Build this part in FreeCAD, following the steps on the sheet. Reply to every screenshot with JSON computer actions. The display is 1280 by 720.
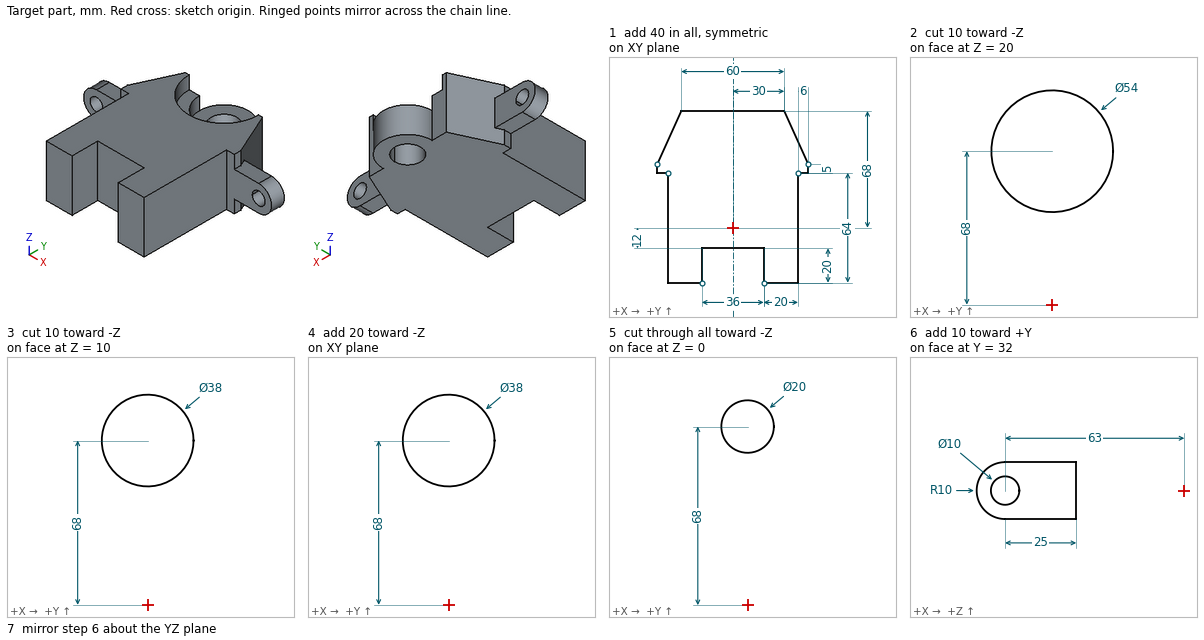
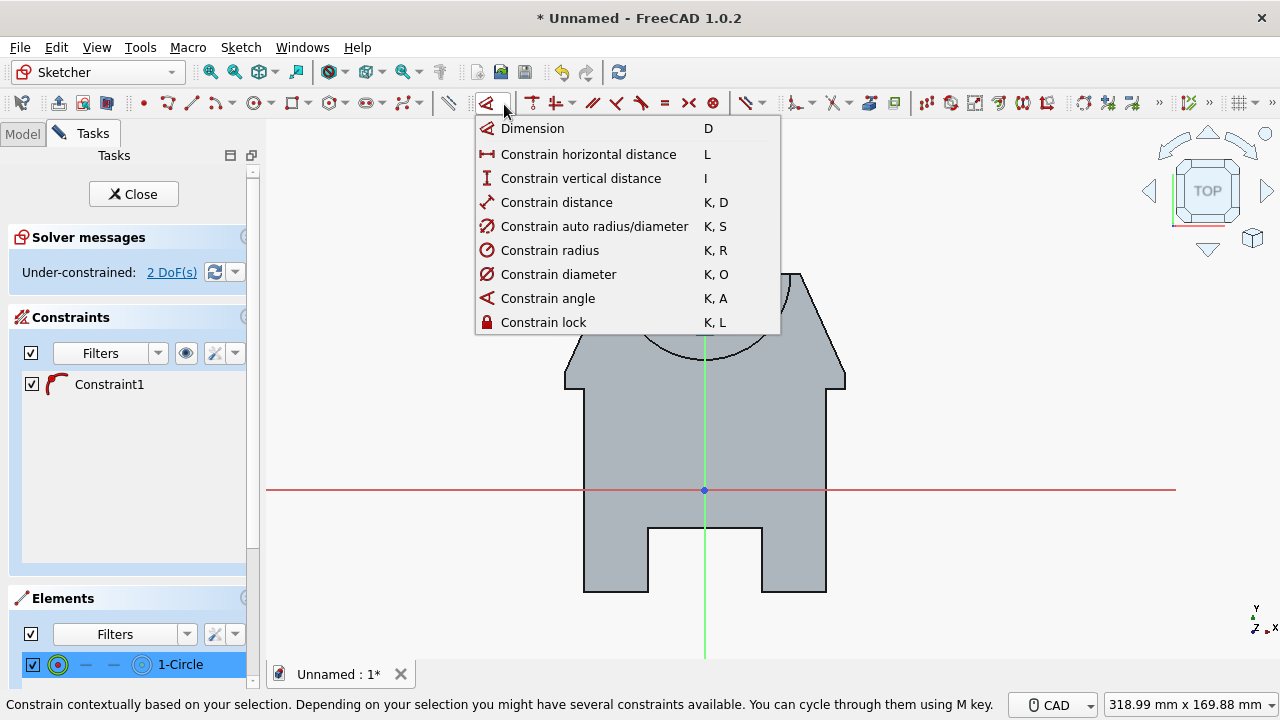
{"action": "left_click", "coordinate": [628, 274]}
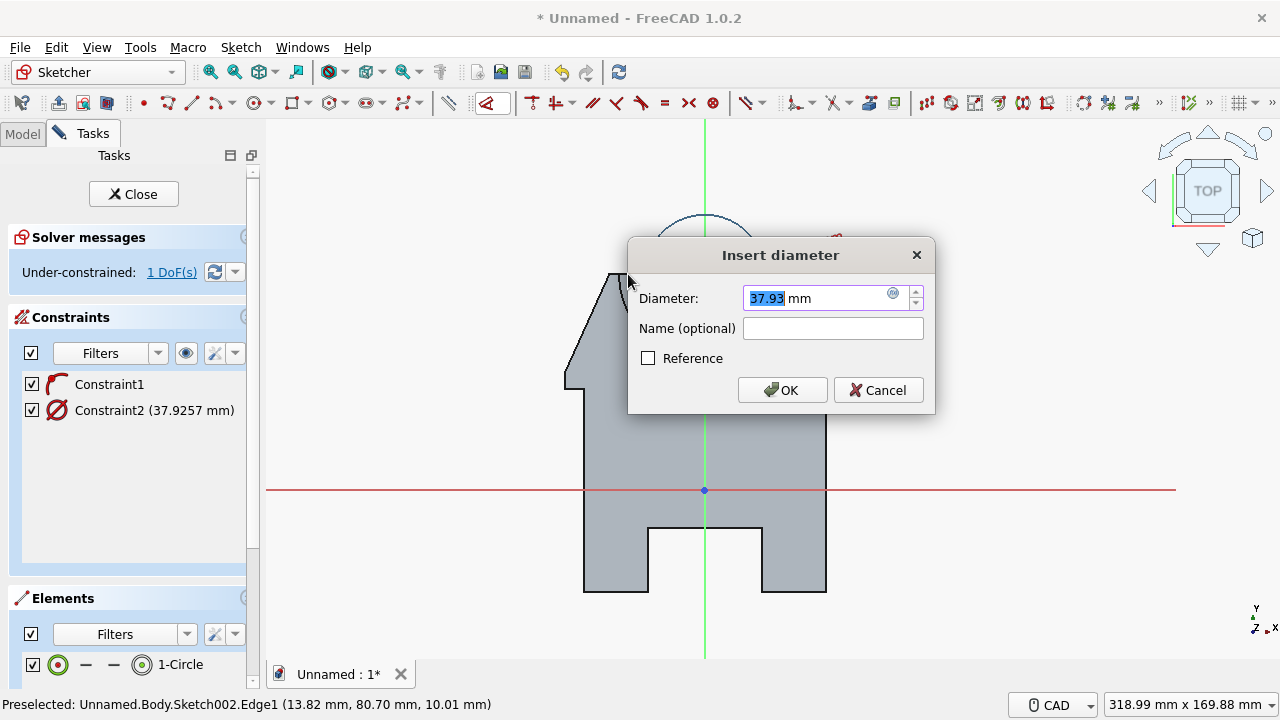
{"action": "type", "text": "38"}
{"action": "key", "text": "Return"}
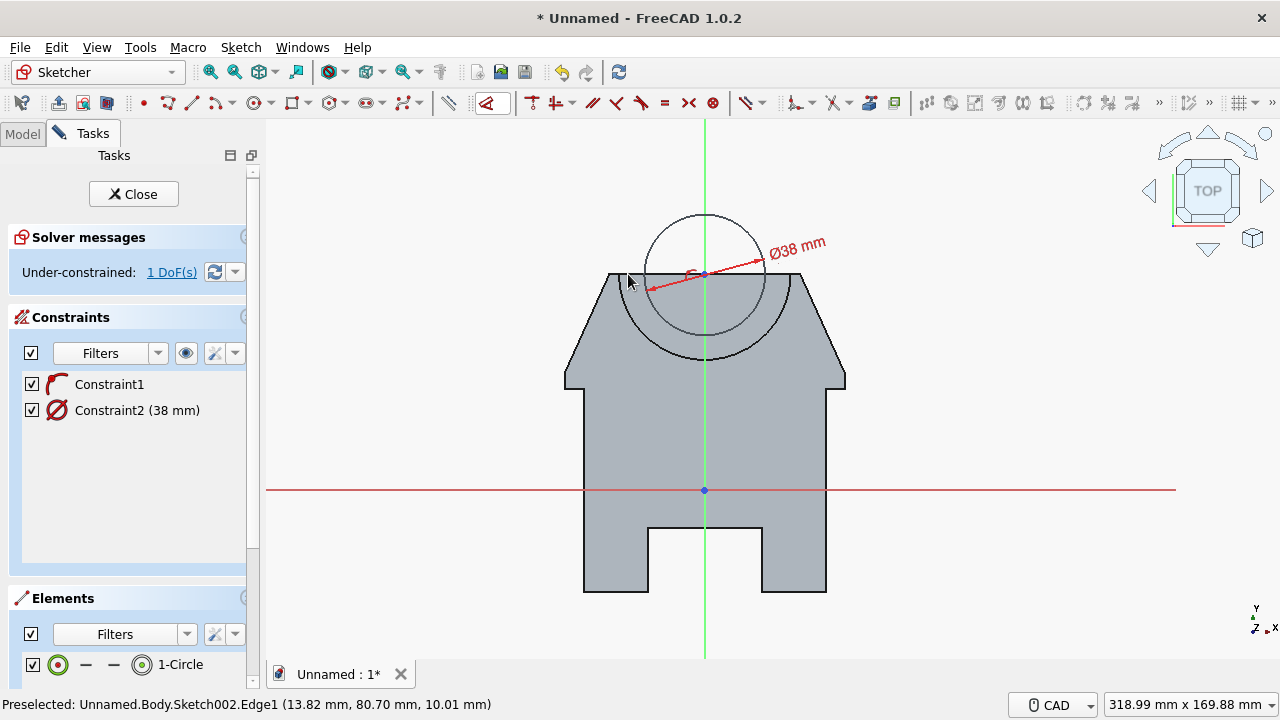
{"action": "left_click", "coordinate": [705, 275]}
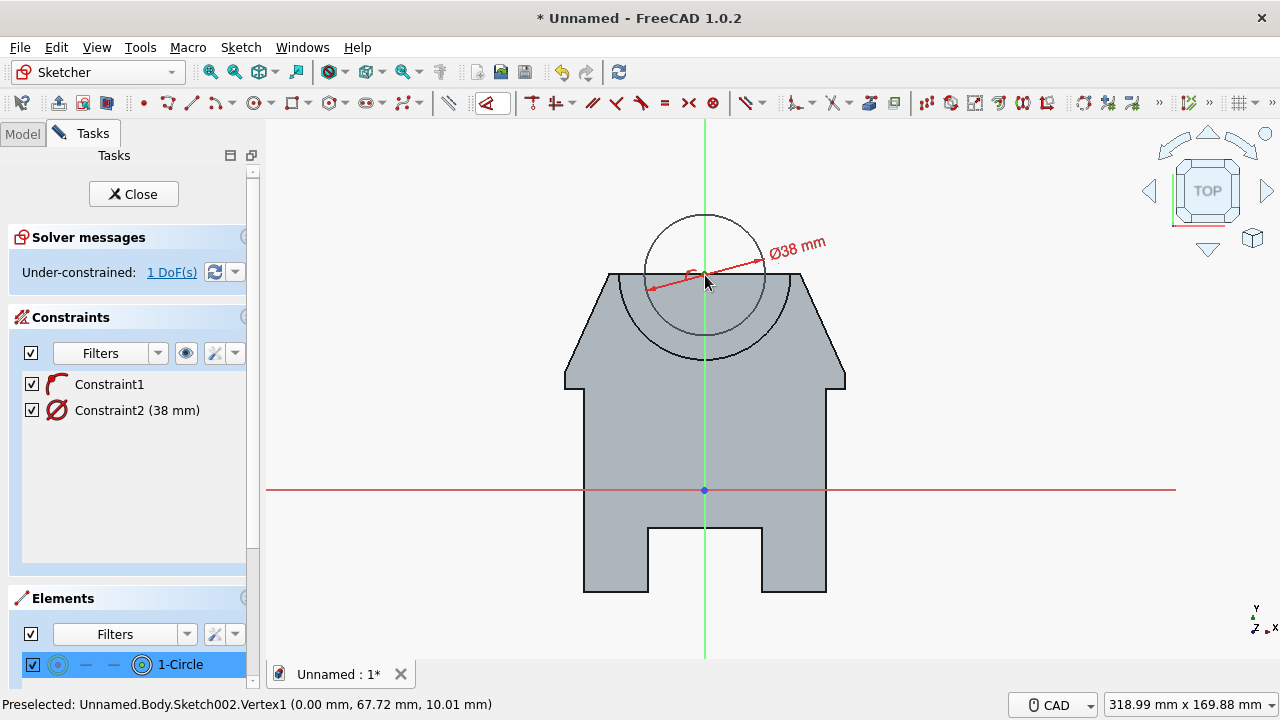
{"action": "key", "text": "i"}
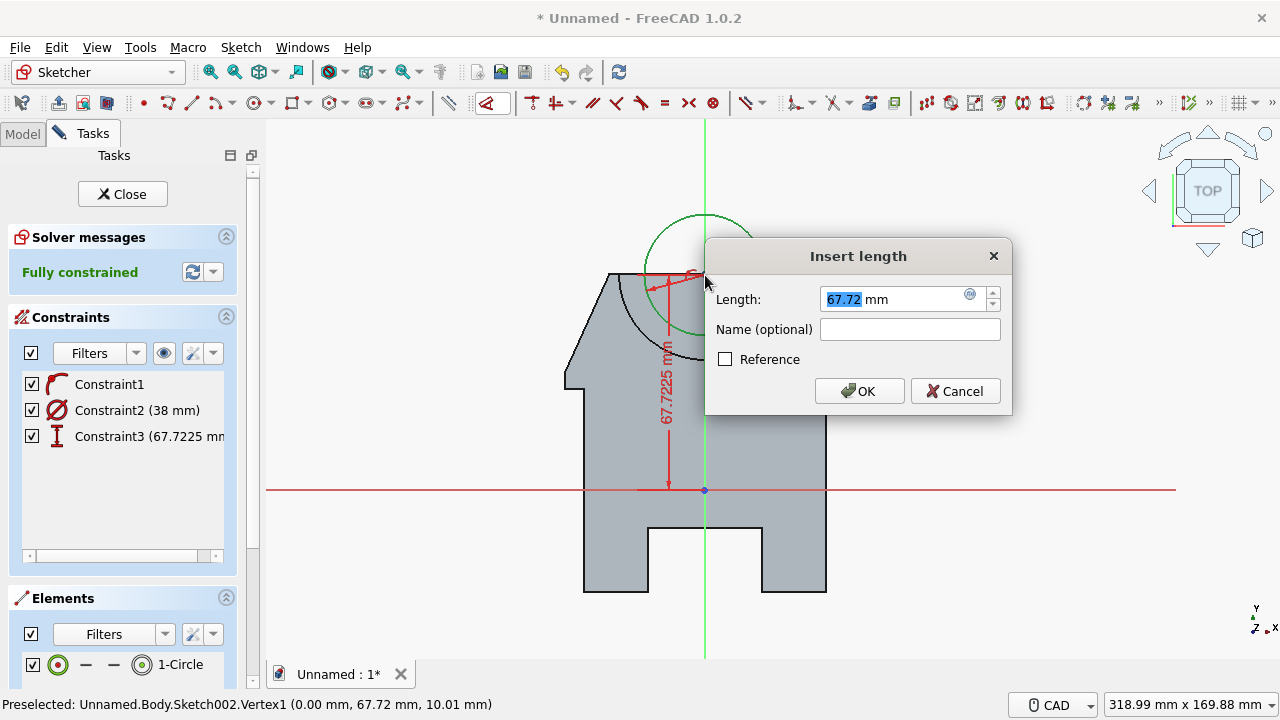
{"action": "type", "text": "68"}
{"action": "key", "text": "Return"}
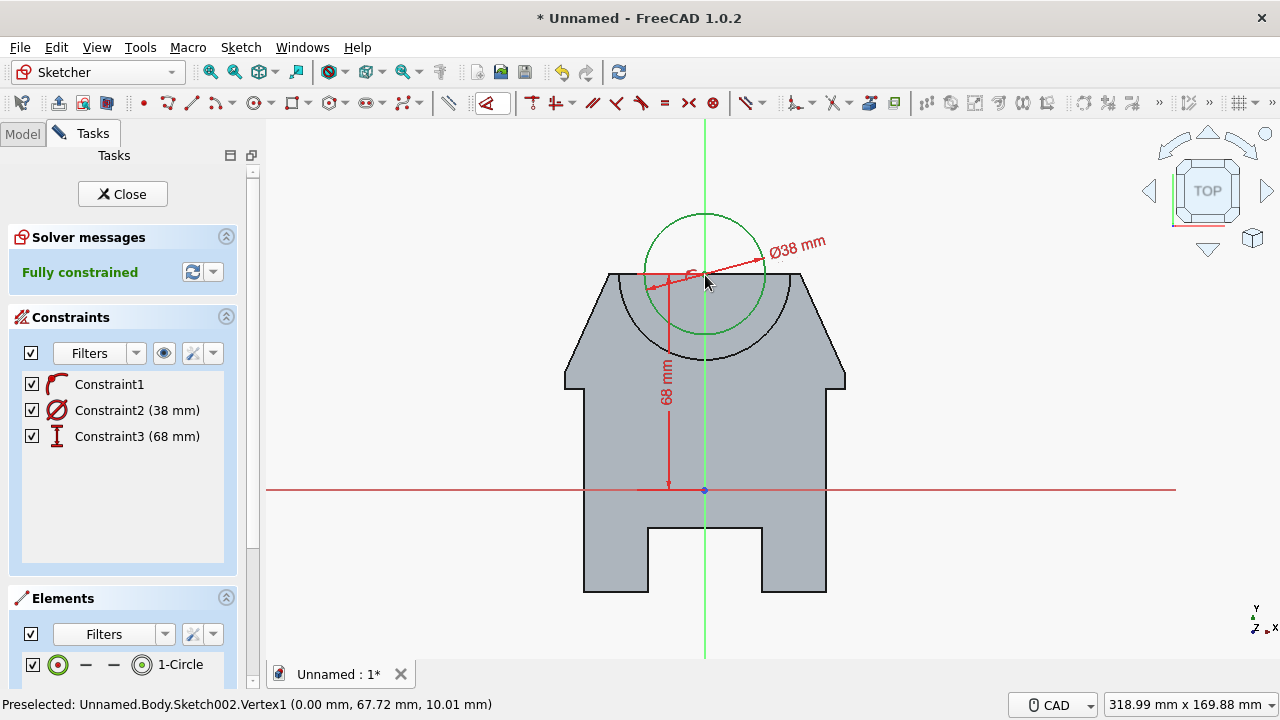
{"action": "left_click", "coordinate": [123, 194]}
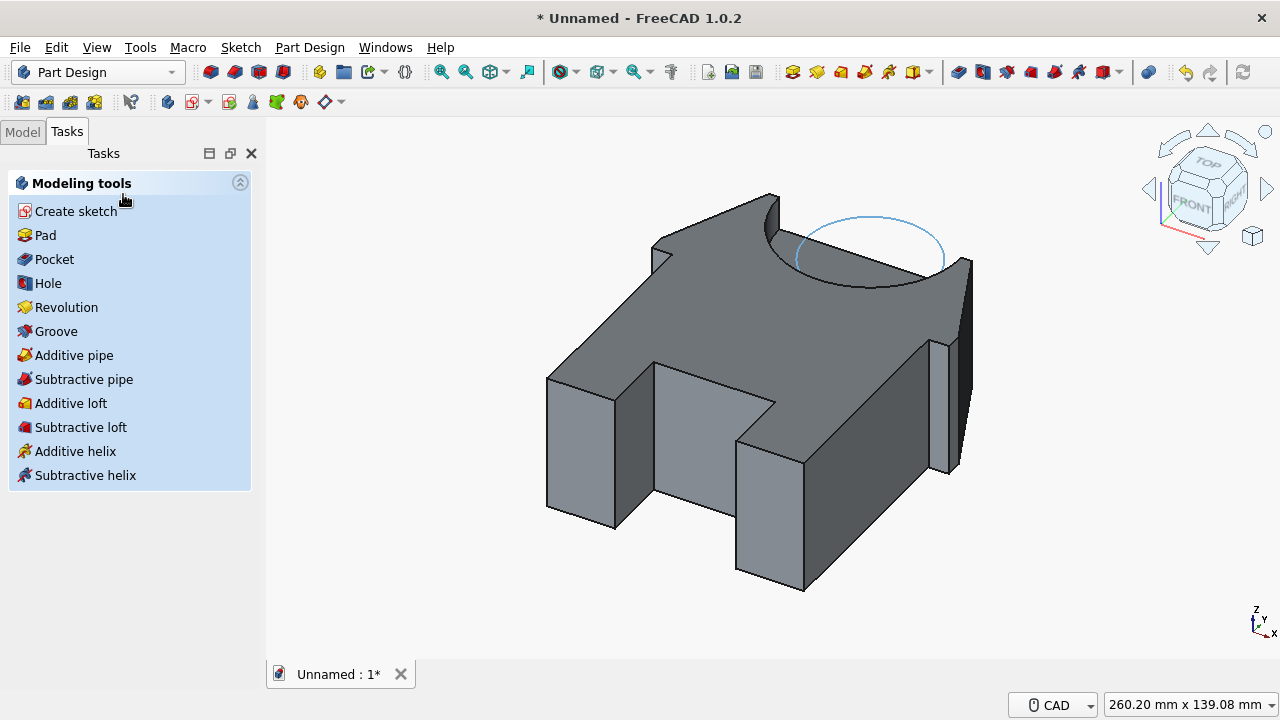
{"action": "left_click", "coordinate": [960, 72]}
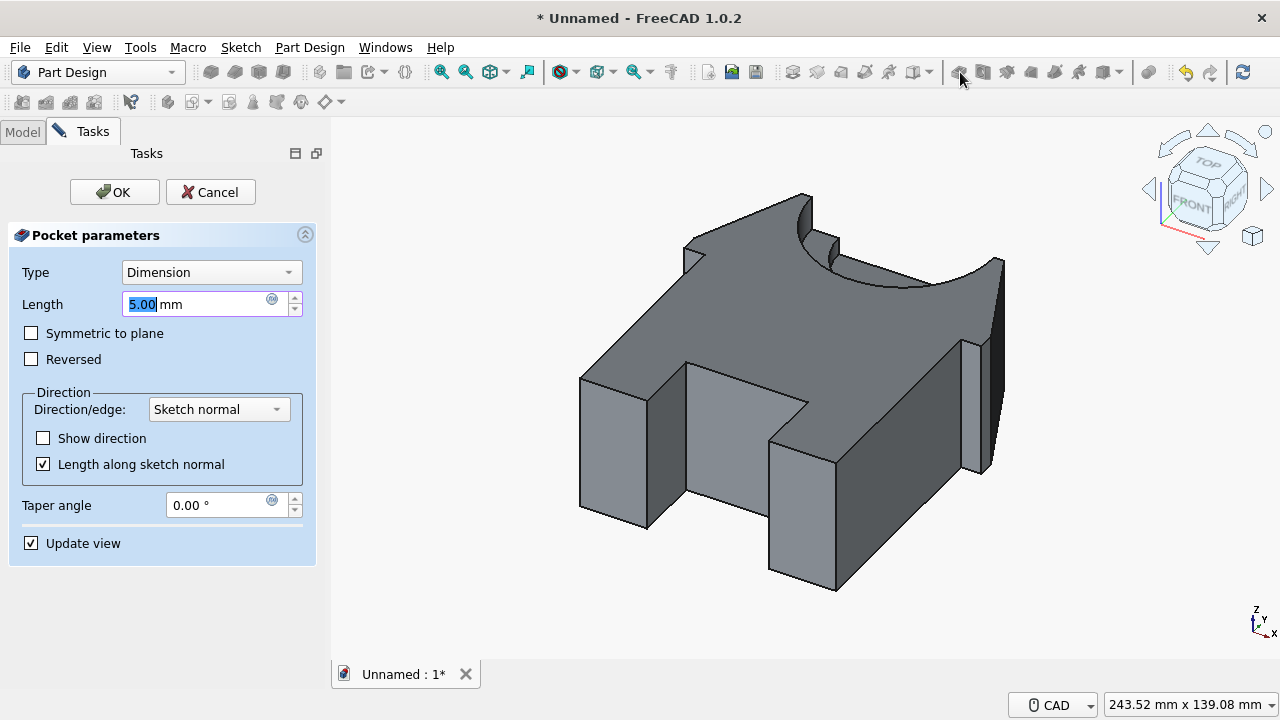
{"action": "type", "text": "10"}
{"action": "key", "text": "Tab"}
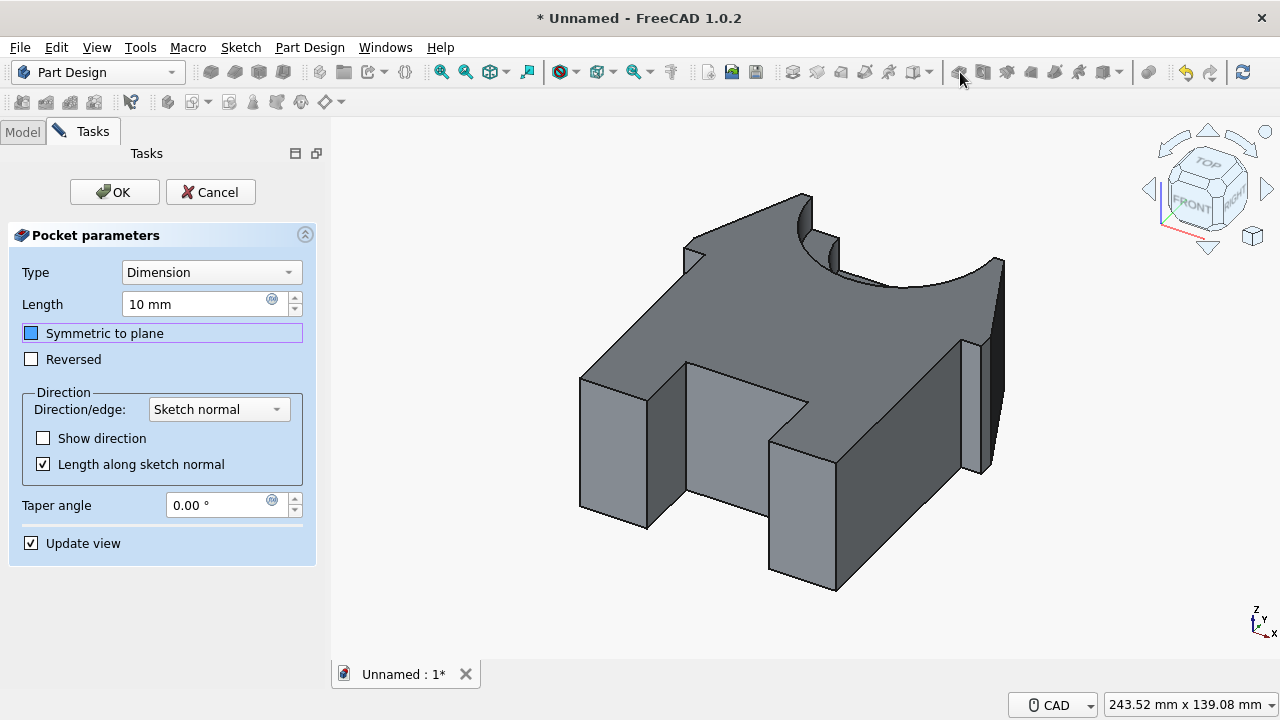
{"action": "left_click", "coordinate": [115, 192]}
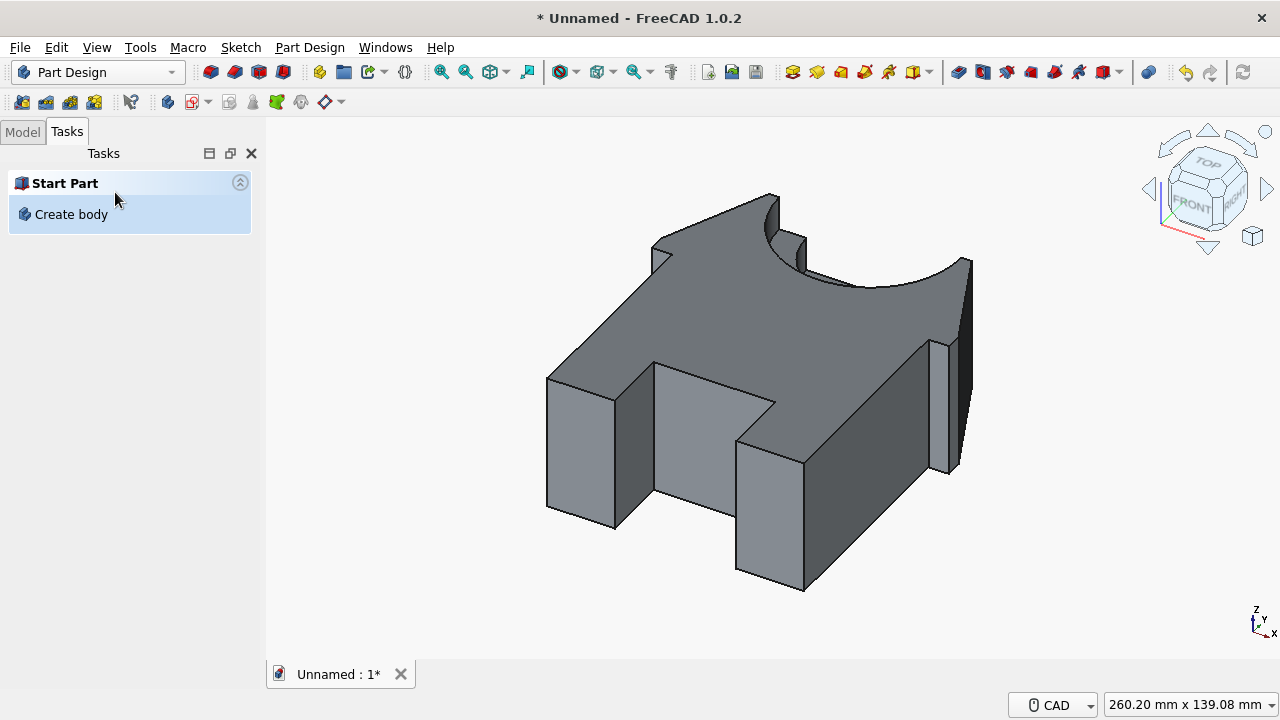
{"action": "left_click", "coordinate": [192, 102]}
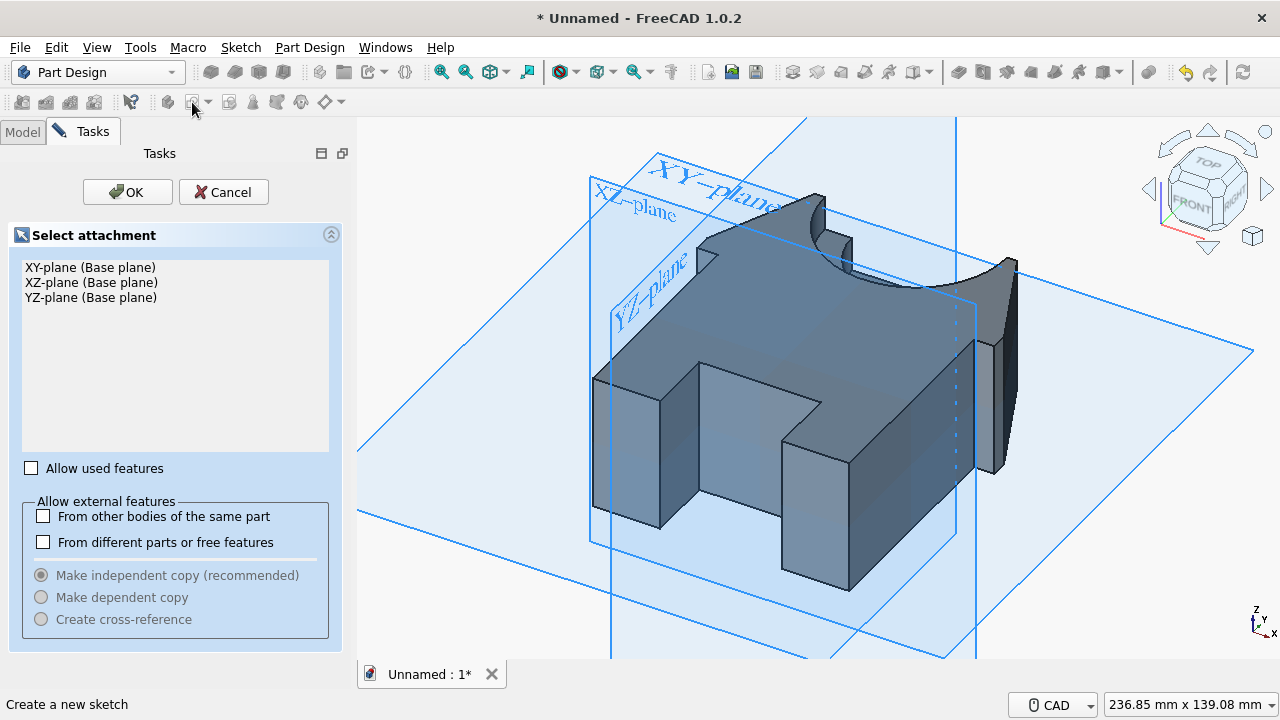
{"action": "left_click", "coordinate": [82, 268]}